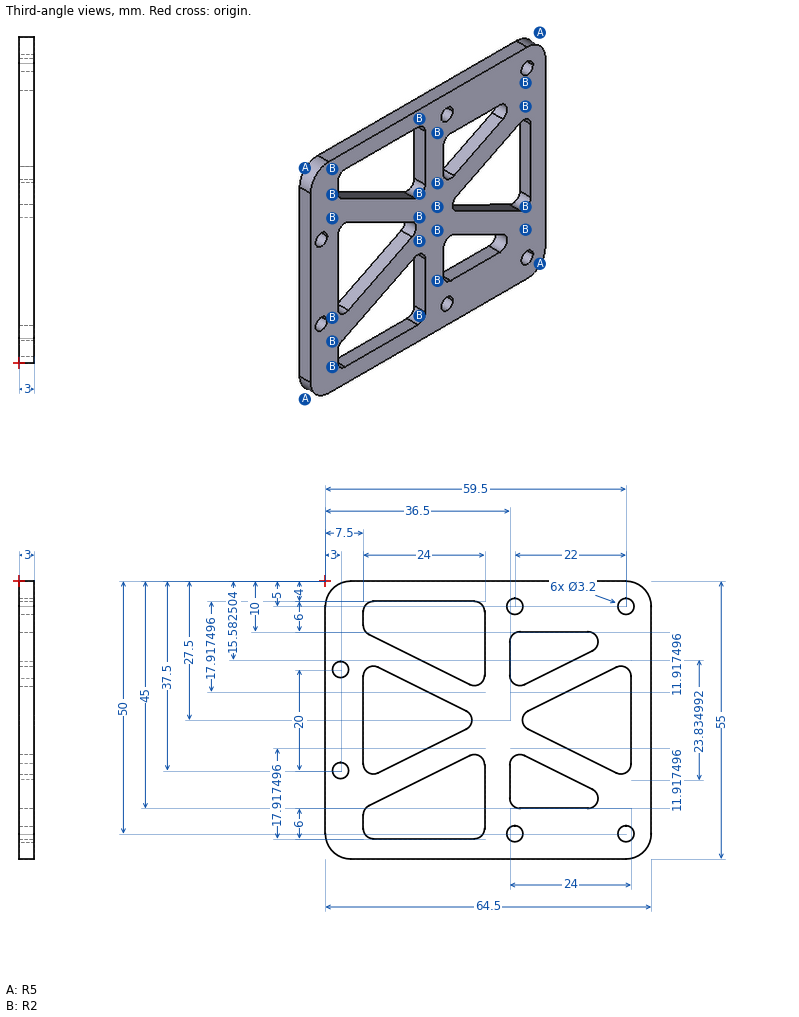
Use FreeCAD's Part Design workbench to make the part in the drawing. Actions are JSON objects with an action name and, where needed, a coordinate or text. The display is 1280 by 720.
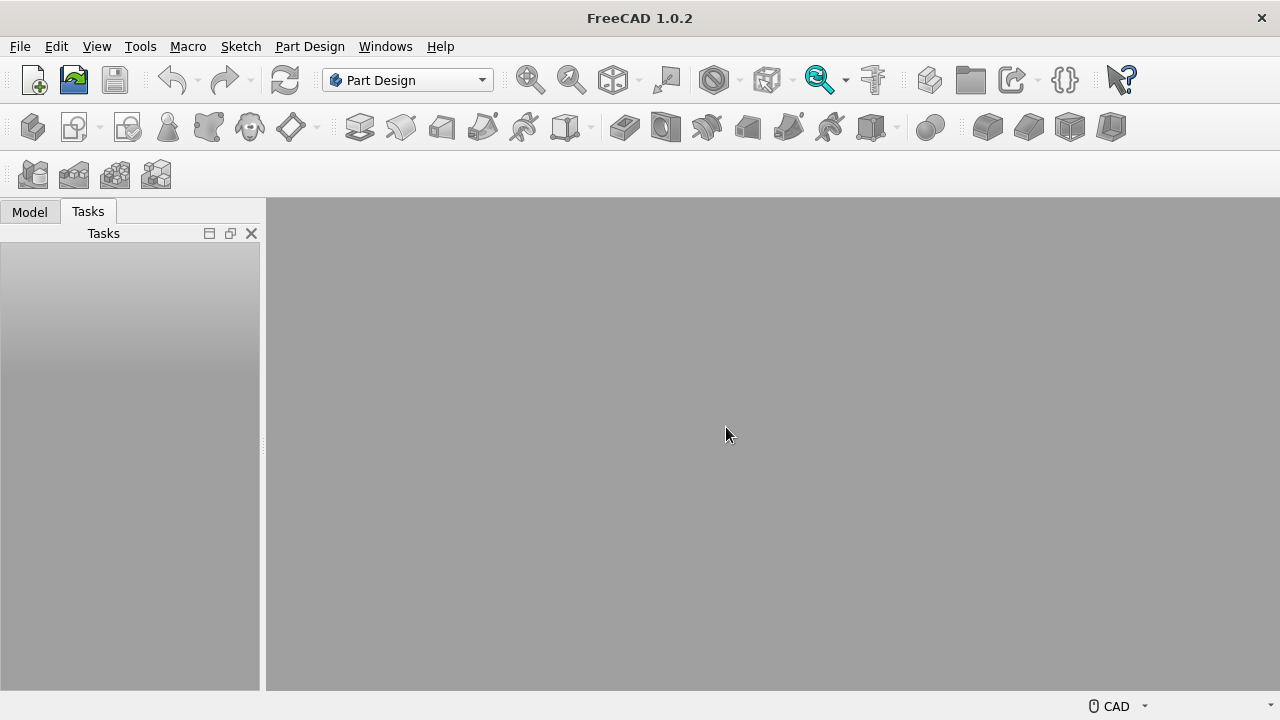
{"action": "left_click", "coordinate": [33, 80]}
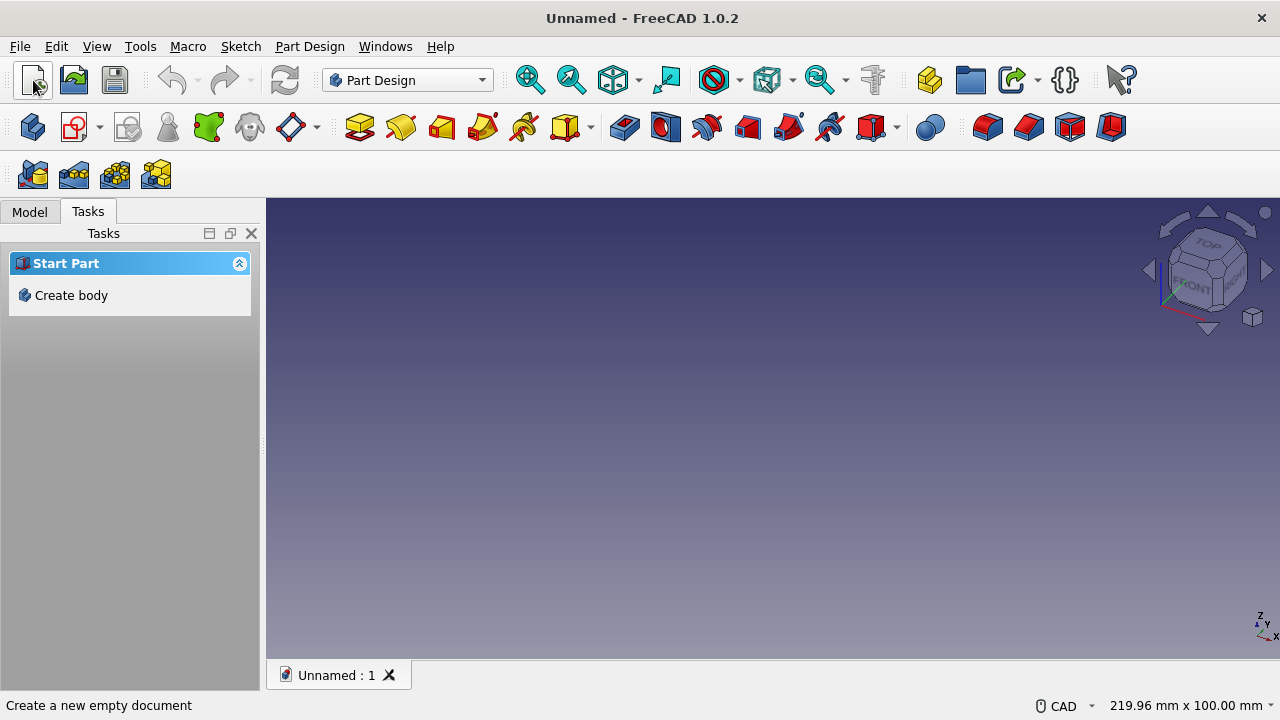
{"action": "left_click", "coordinate": [74, 128]}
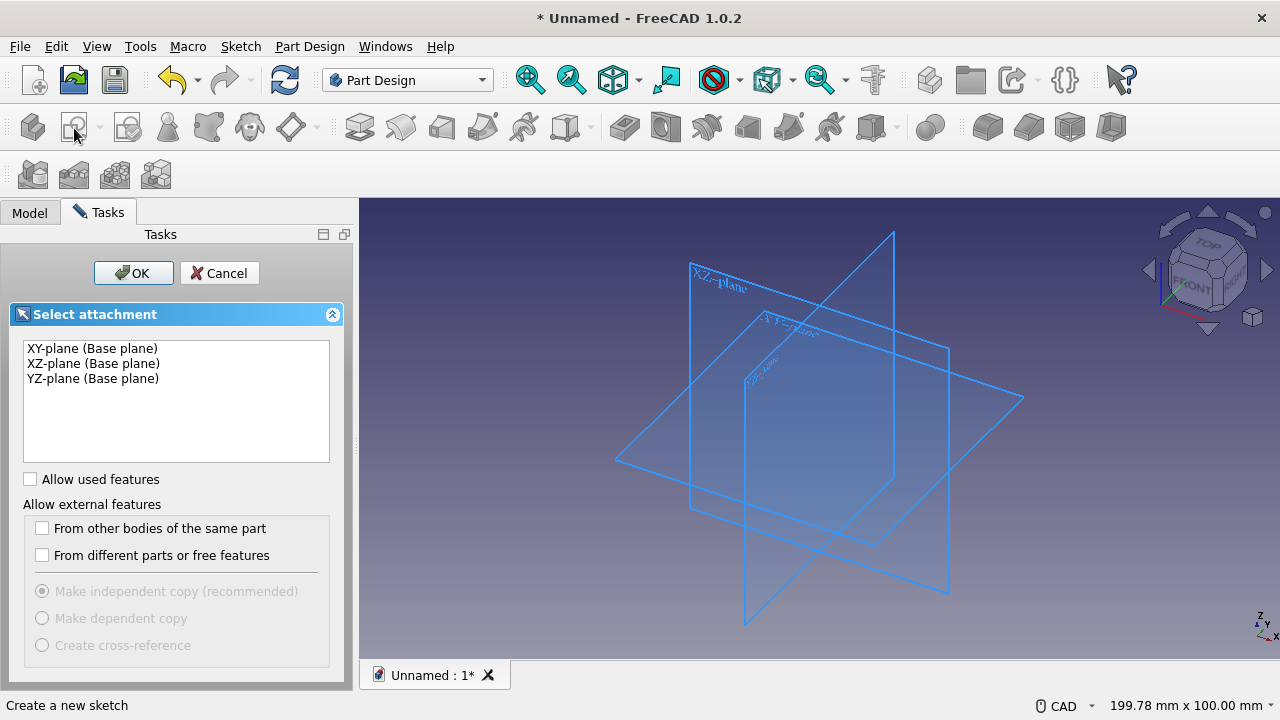
{"action": "left_click", "coordinate": [84, 378]}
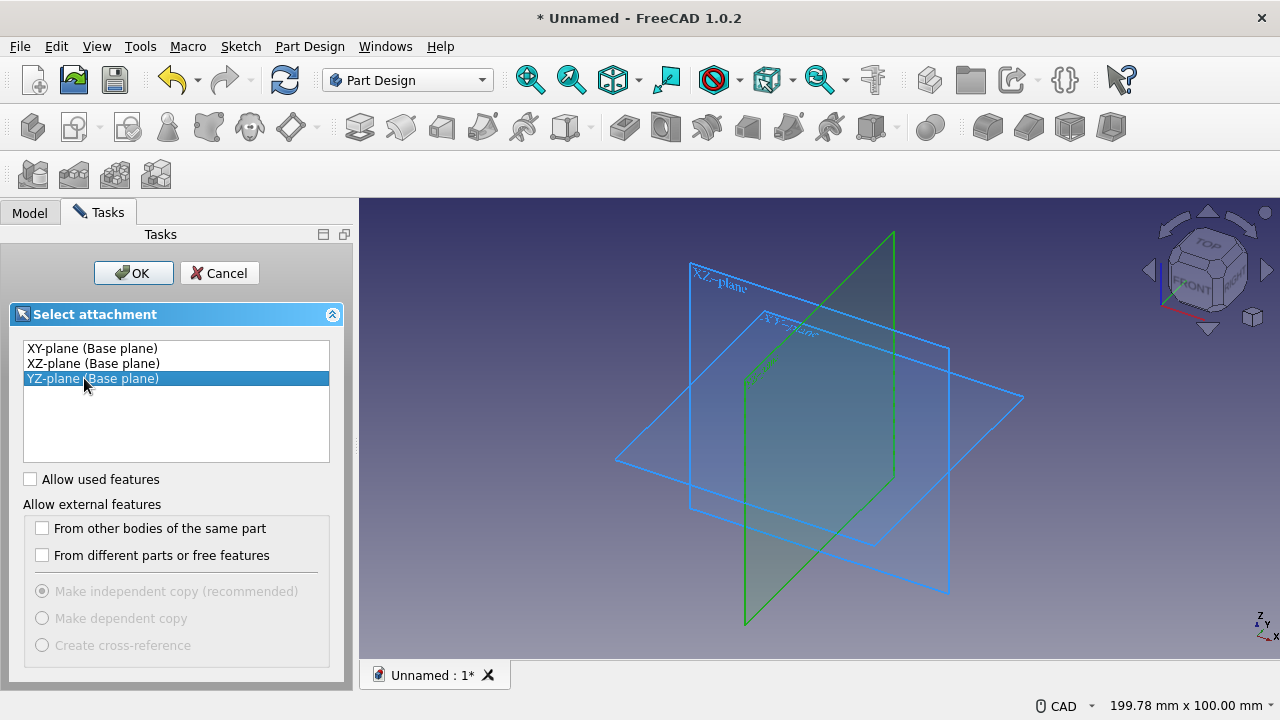
{"action": "left_click", "coordinate": [134, 273]}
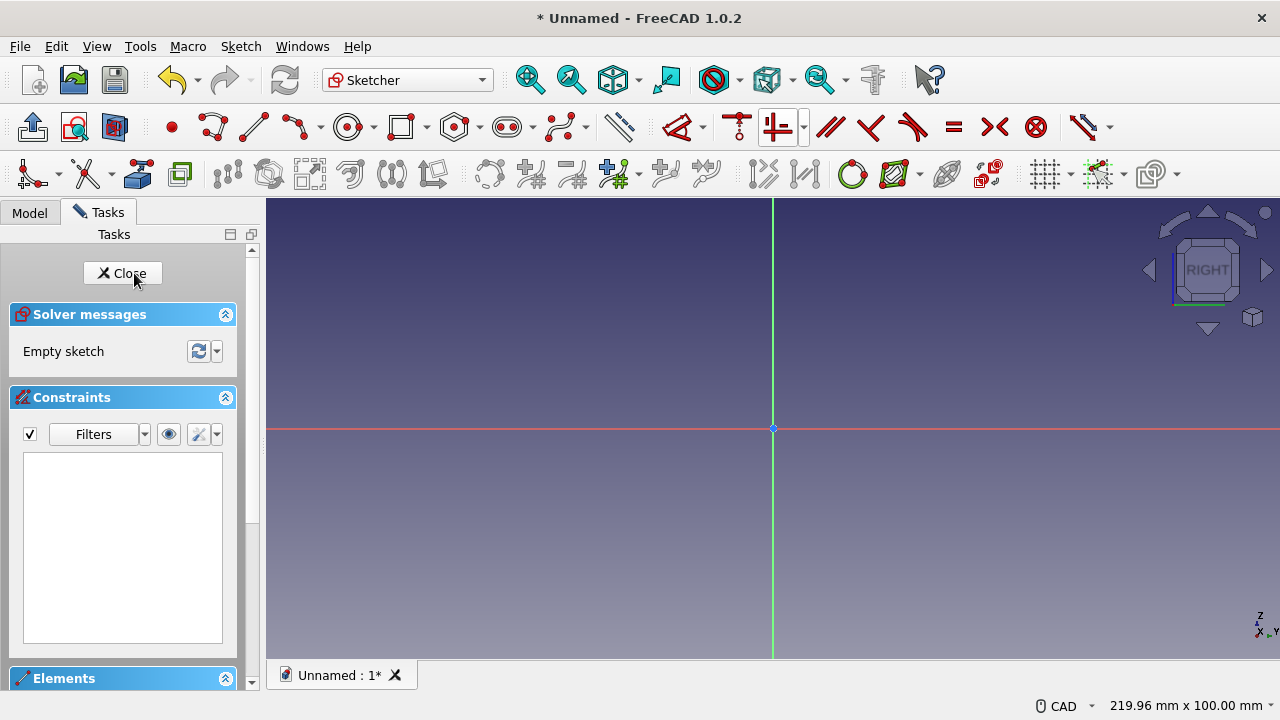
{"action": "scroll", "coordinate": [294, 226], "scroll_direction": "down", "scroll_amount": 1}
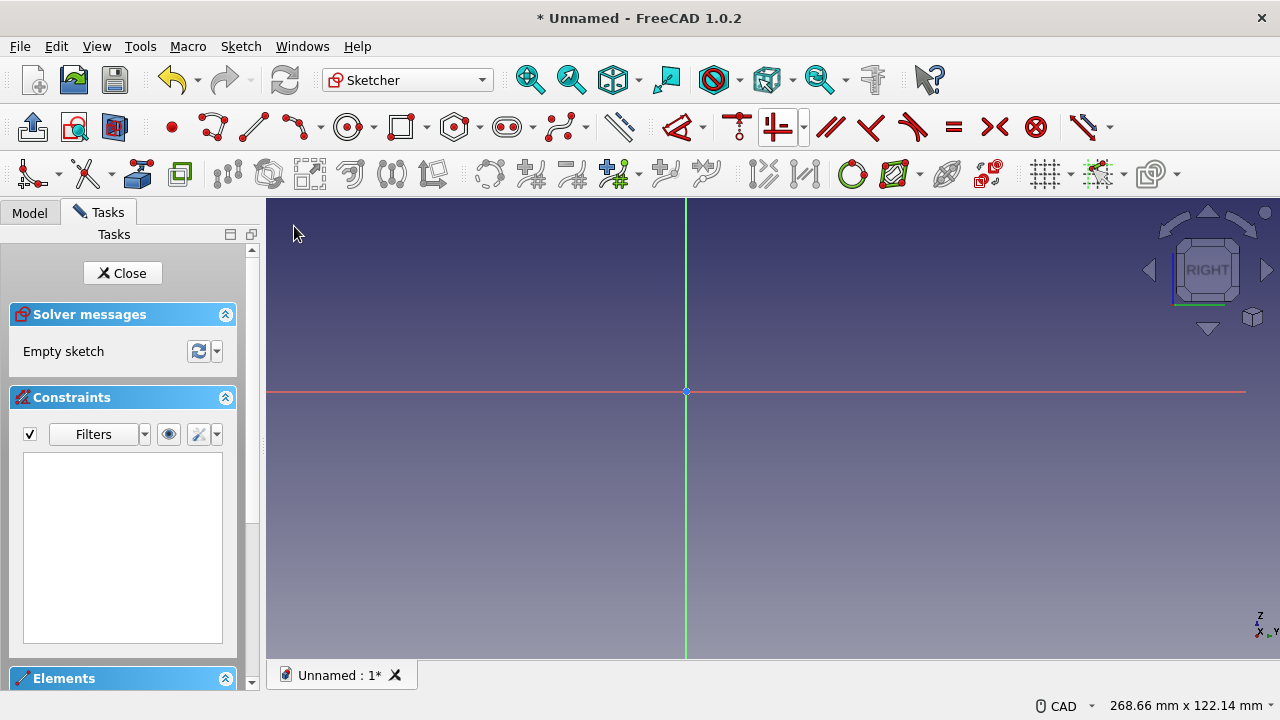
{"action": "scroll", "coordinate": [1018, 631], "scroll_direction": "up", "scroll_amount": 2}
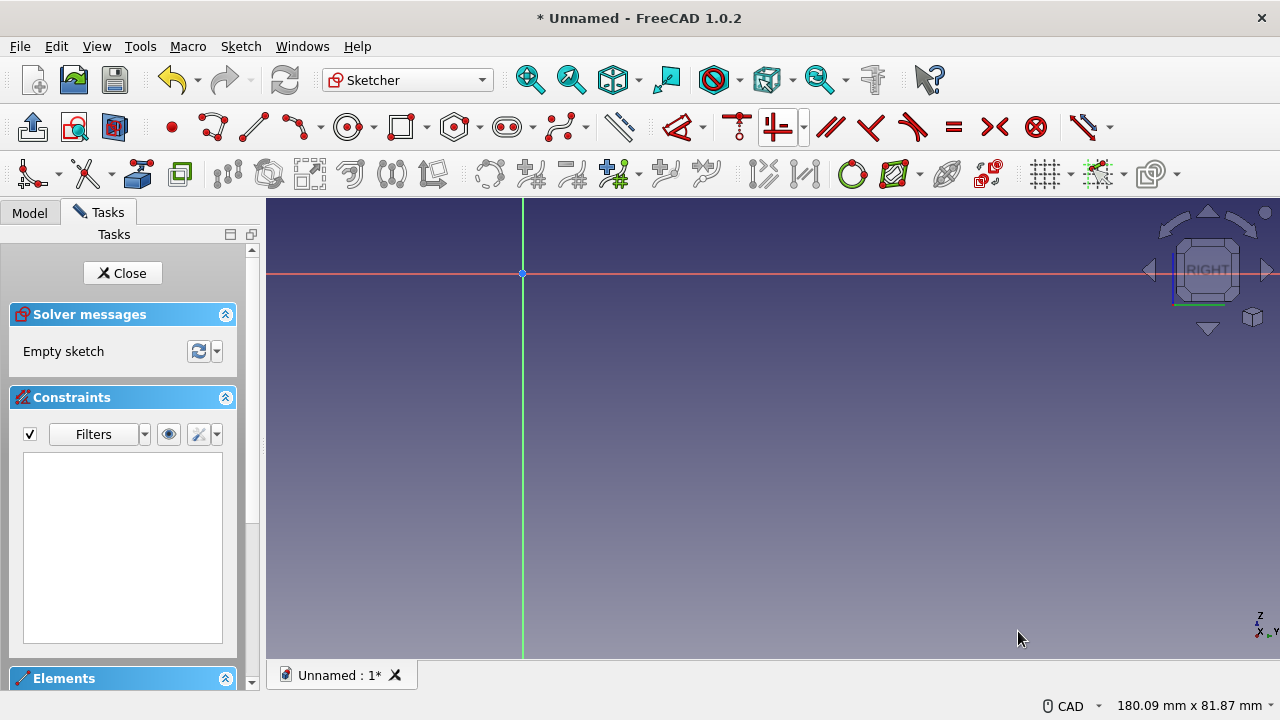
{"action": "left_click", "coordinate": [400, 128]}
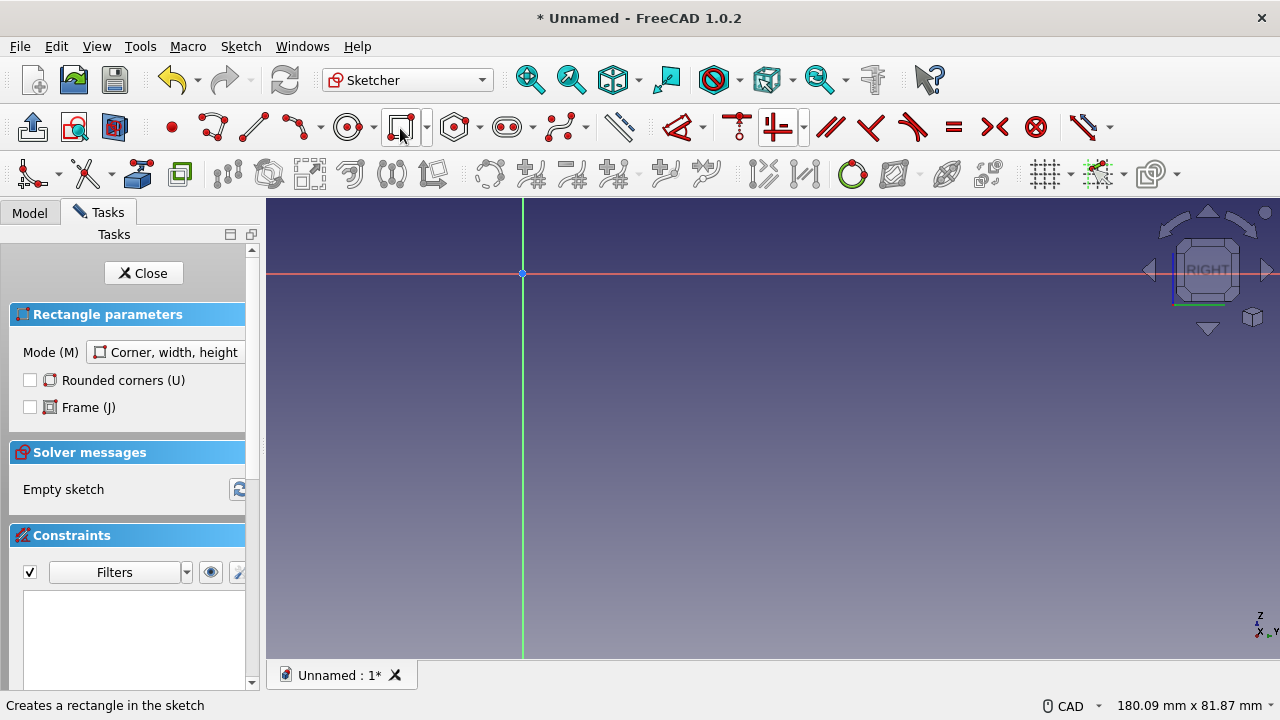
{"action": "left_click", "coordinate": [523, 274]}
{"action": "mouse_move", "coordinate": [886, 583]}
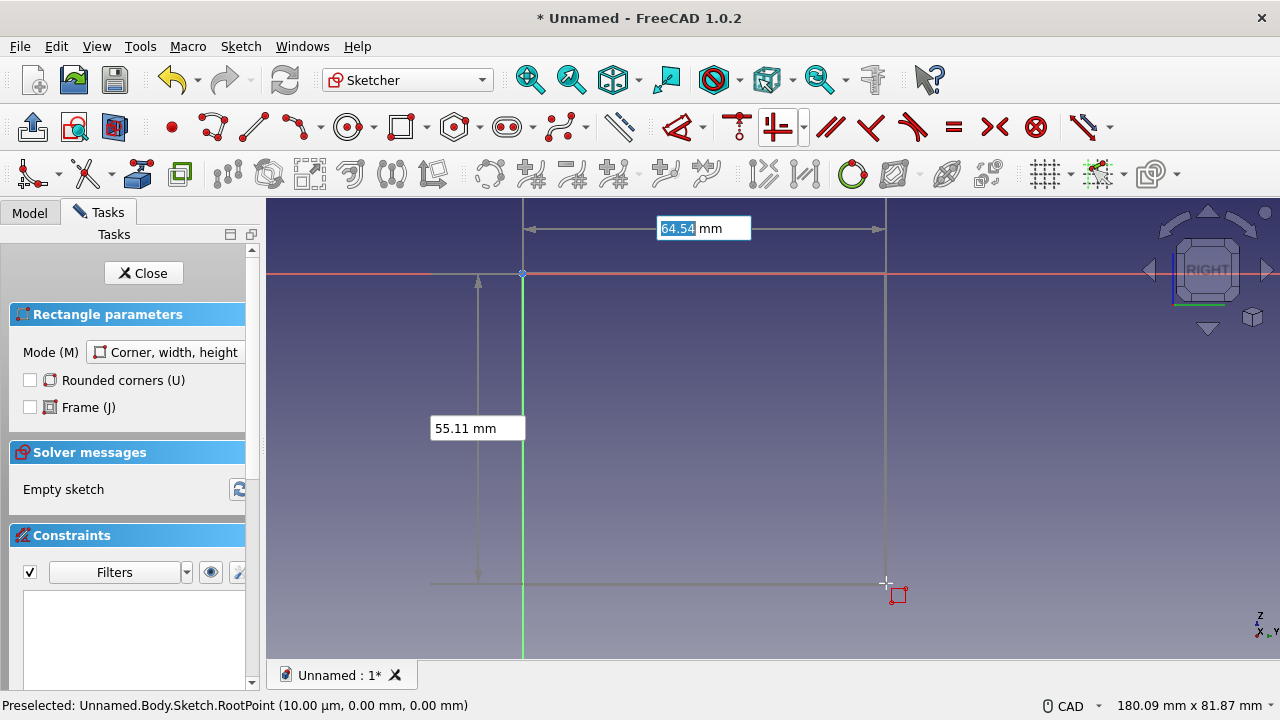
{"action": "type", "text": "64.5"}
{"action": "key", "text": "Tab"}
{"action": "type", "text": "55"}
{"action": "key", "text": "Return"}
{"action": "key", "text": "Escape"}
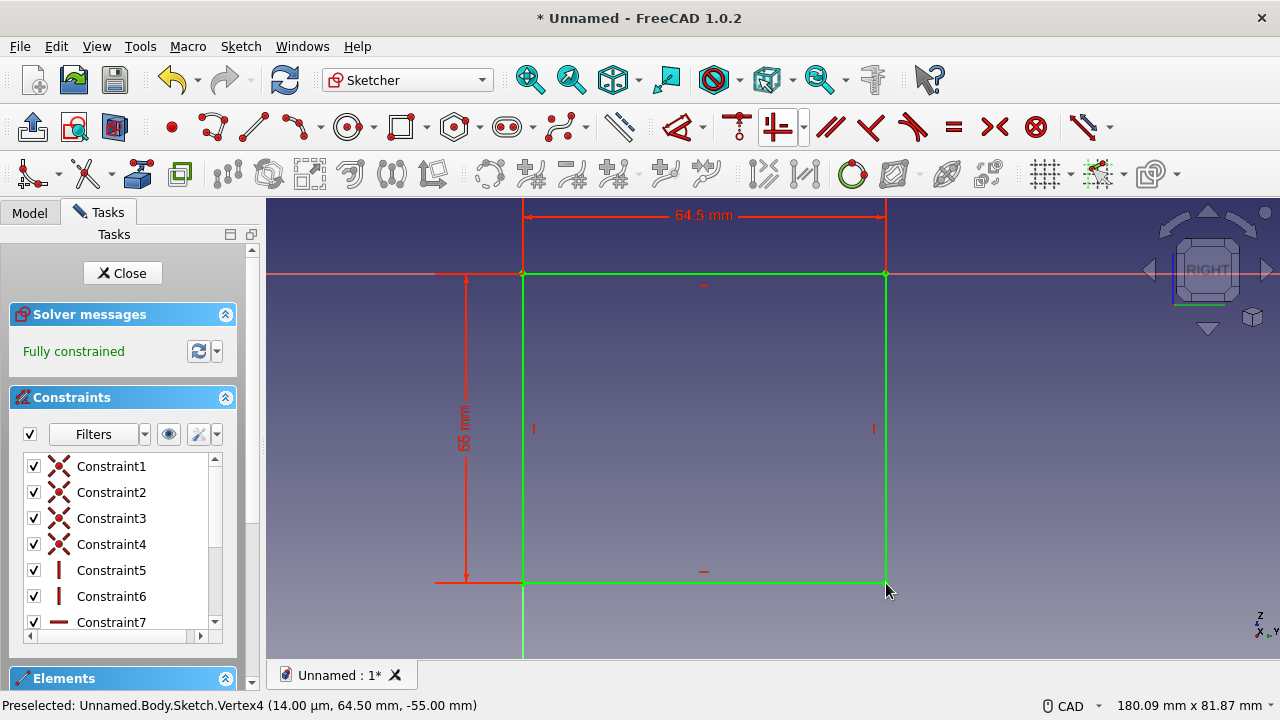
{"action": "left_click", "coordinate": [123, 273]}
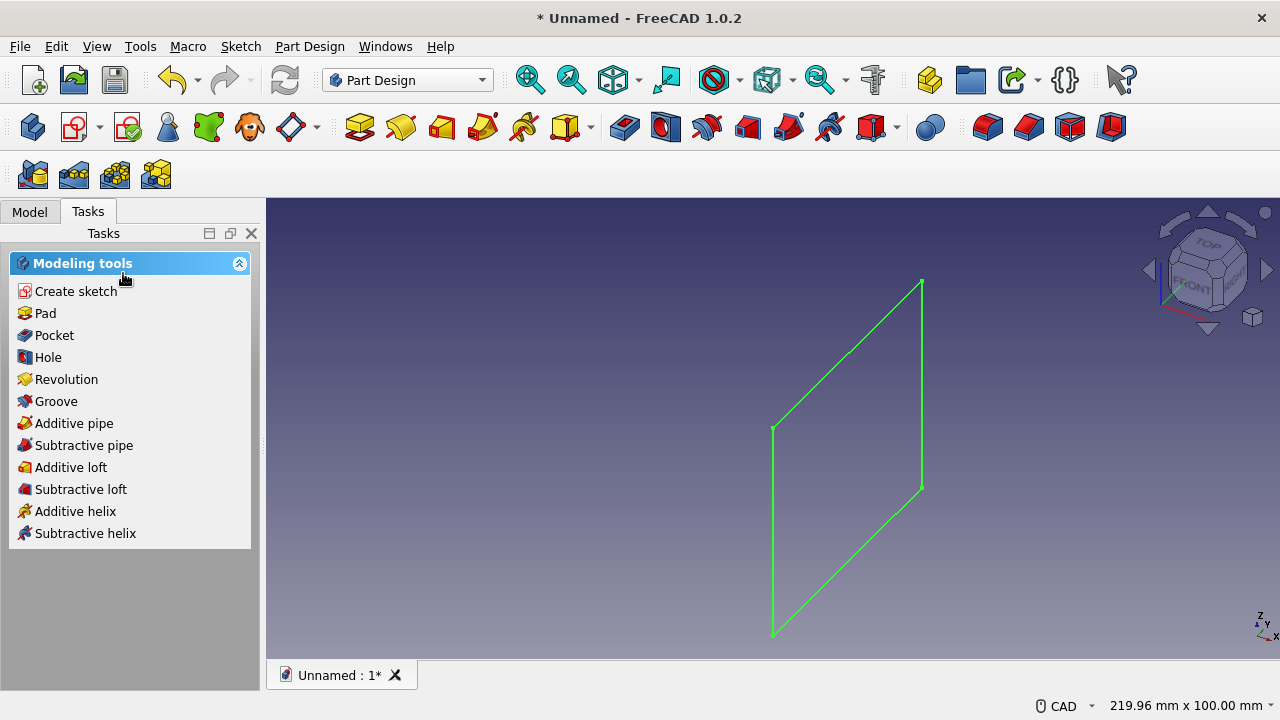
{"action": "left_click", "coordinate": [360, 128]}